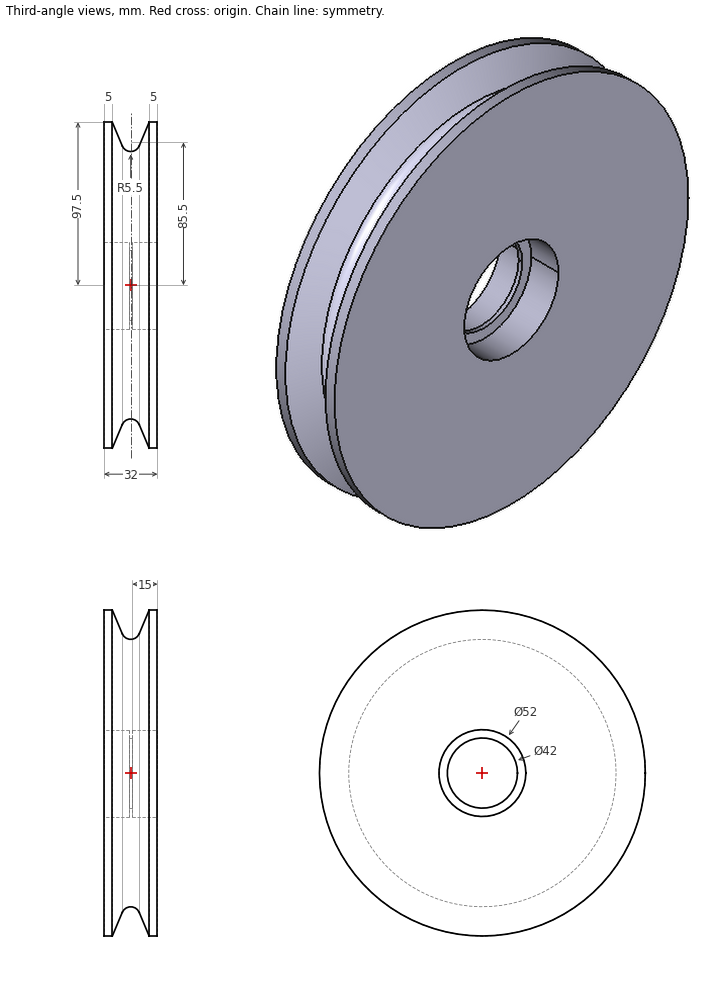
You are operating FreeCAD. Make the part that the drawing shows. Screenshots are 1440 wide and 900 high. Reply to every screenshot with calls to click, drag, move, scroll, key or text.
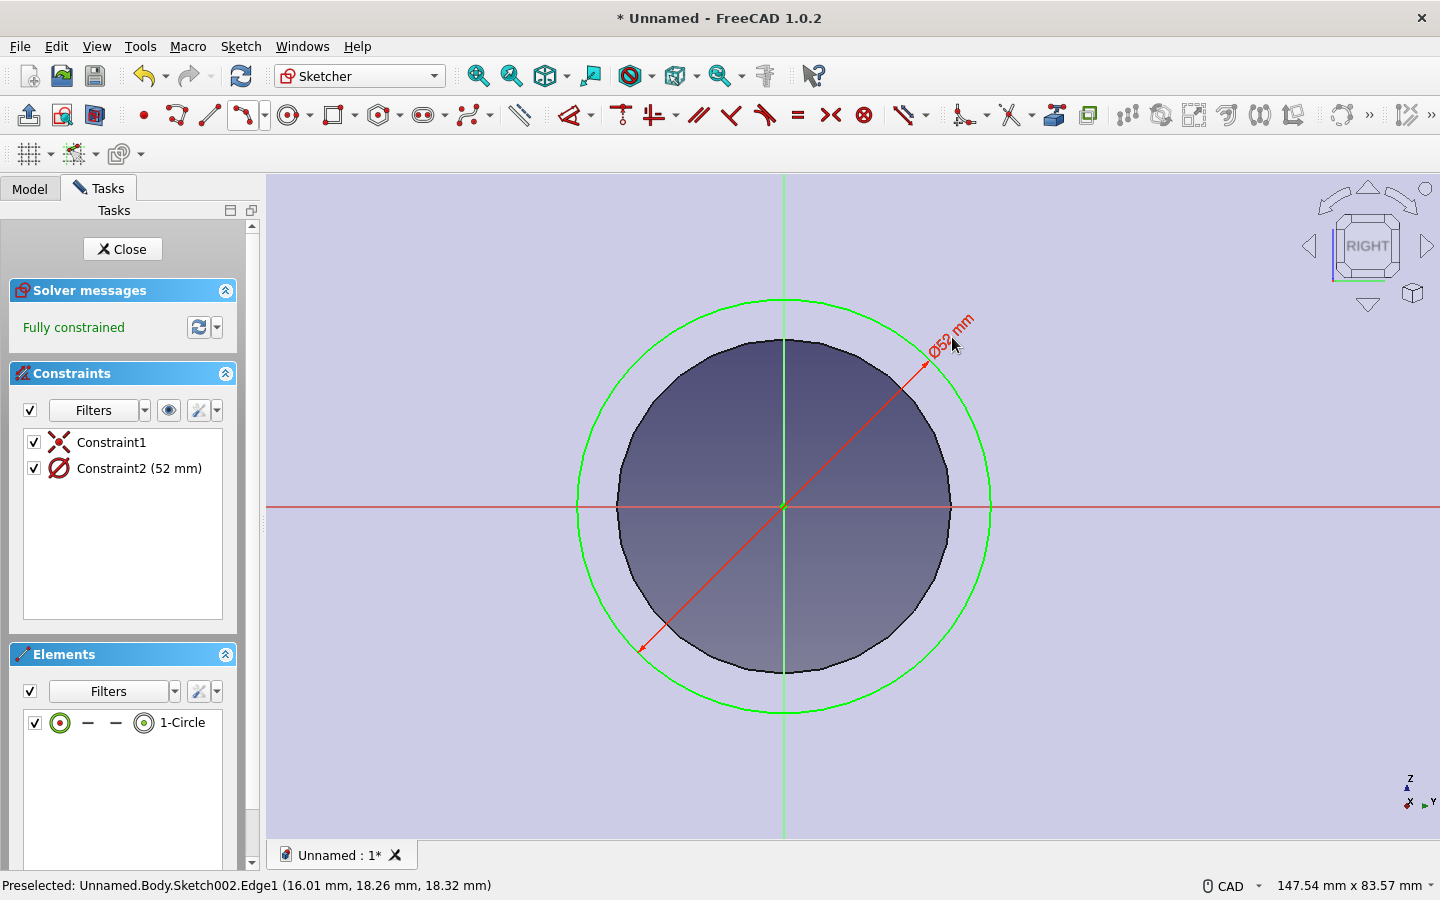
click(123, 249)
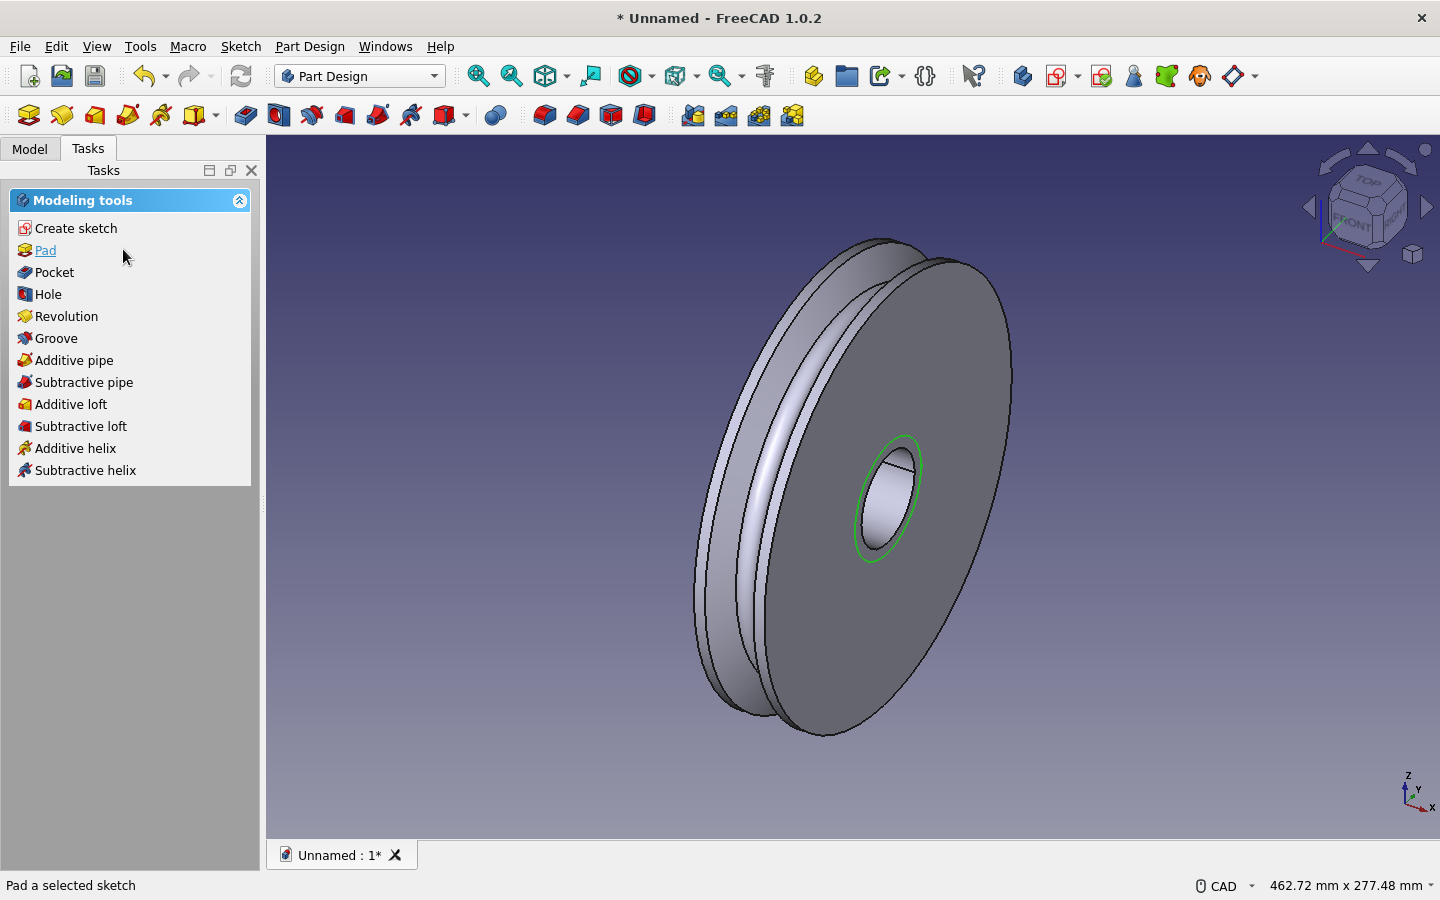
click(246, 116)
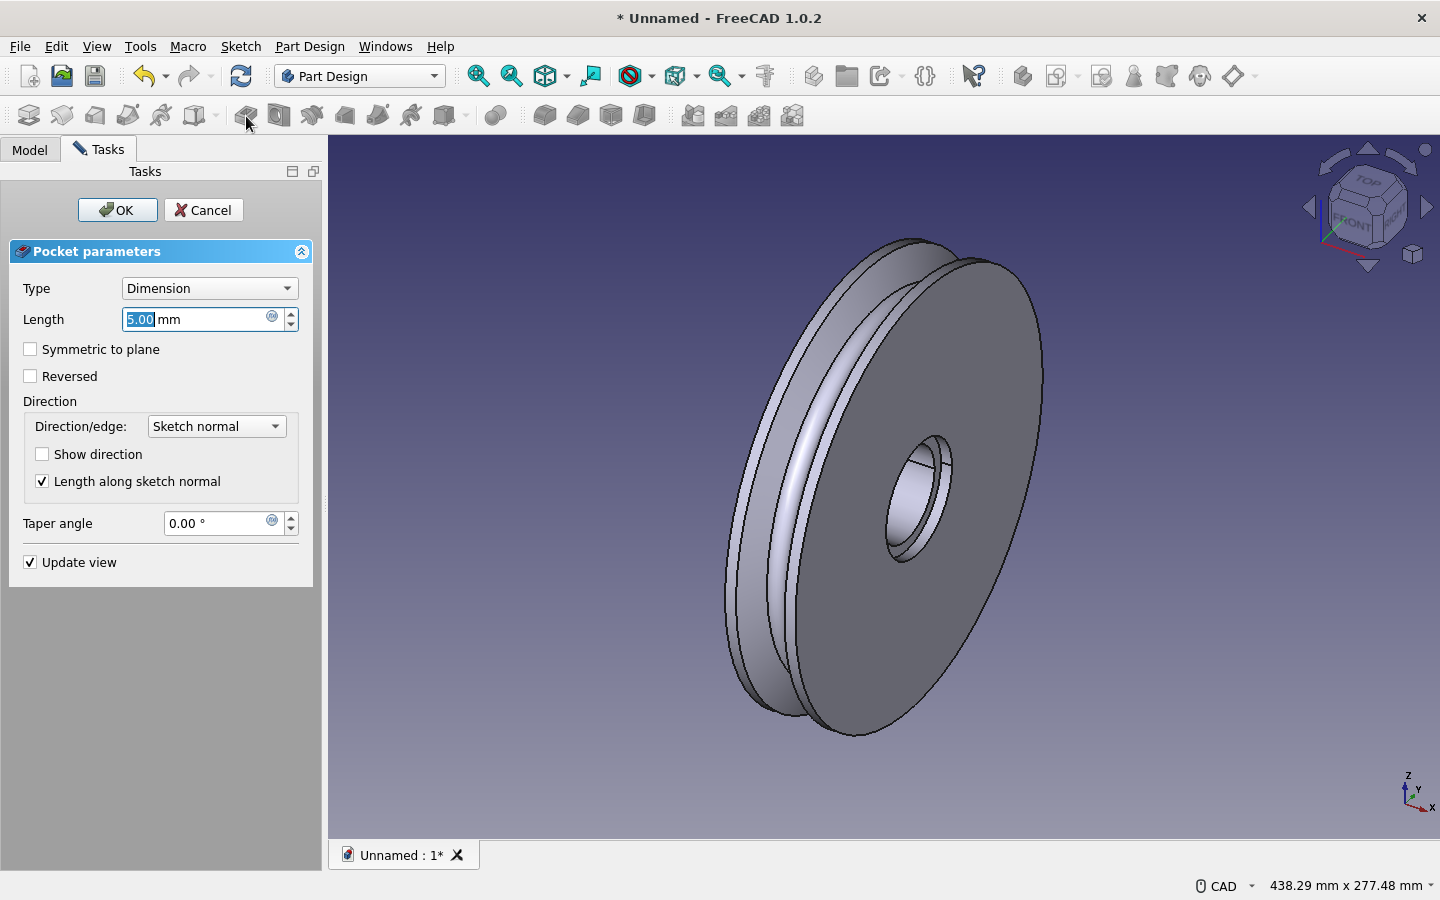
text(15)
key(Tab)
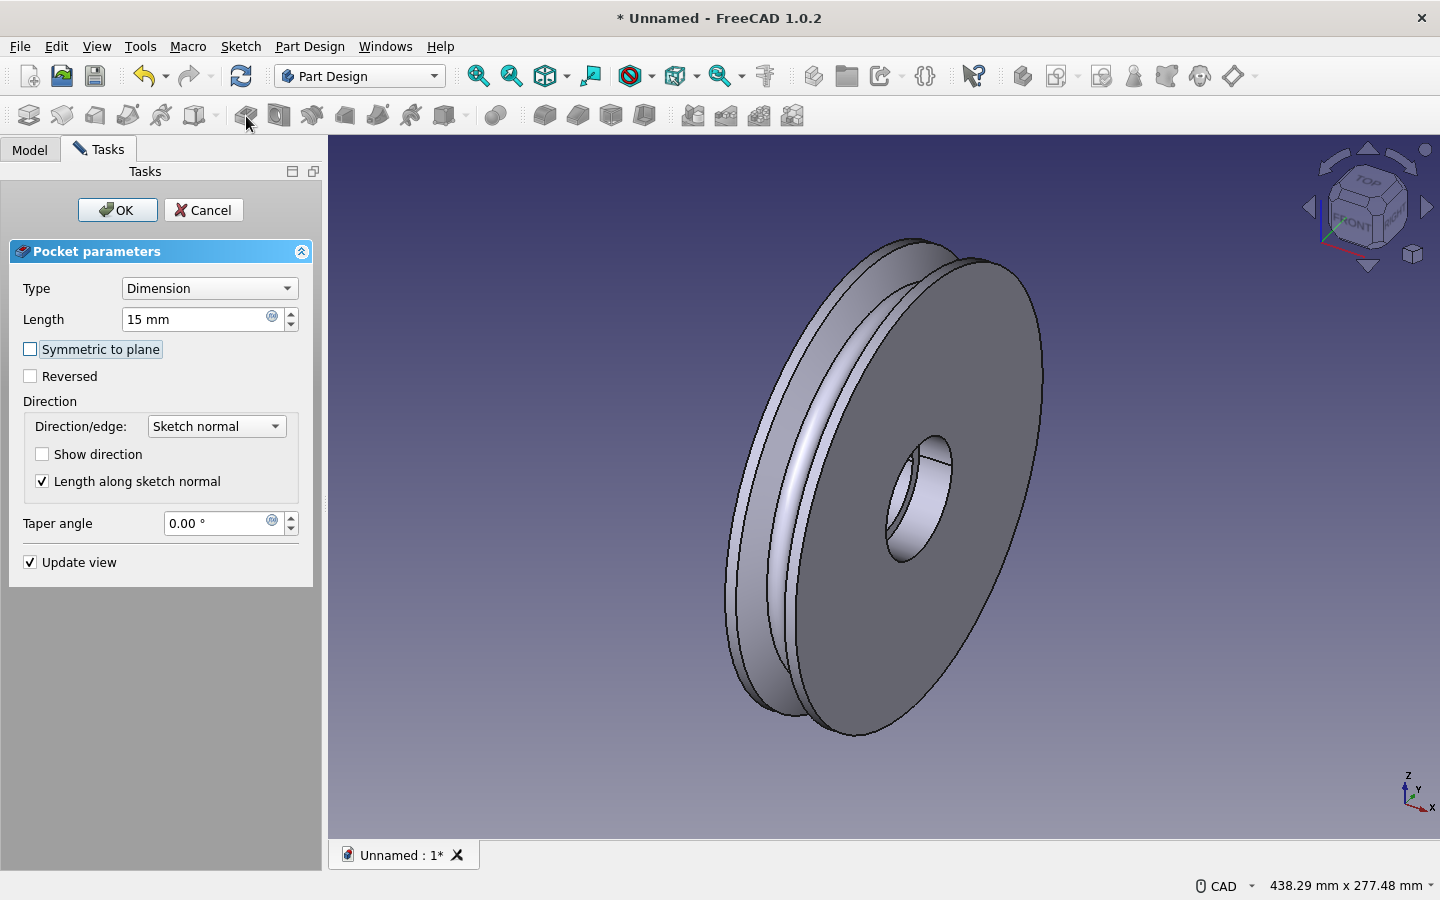
click(118, 210)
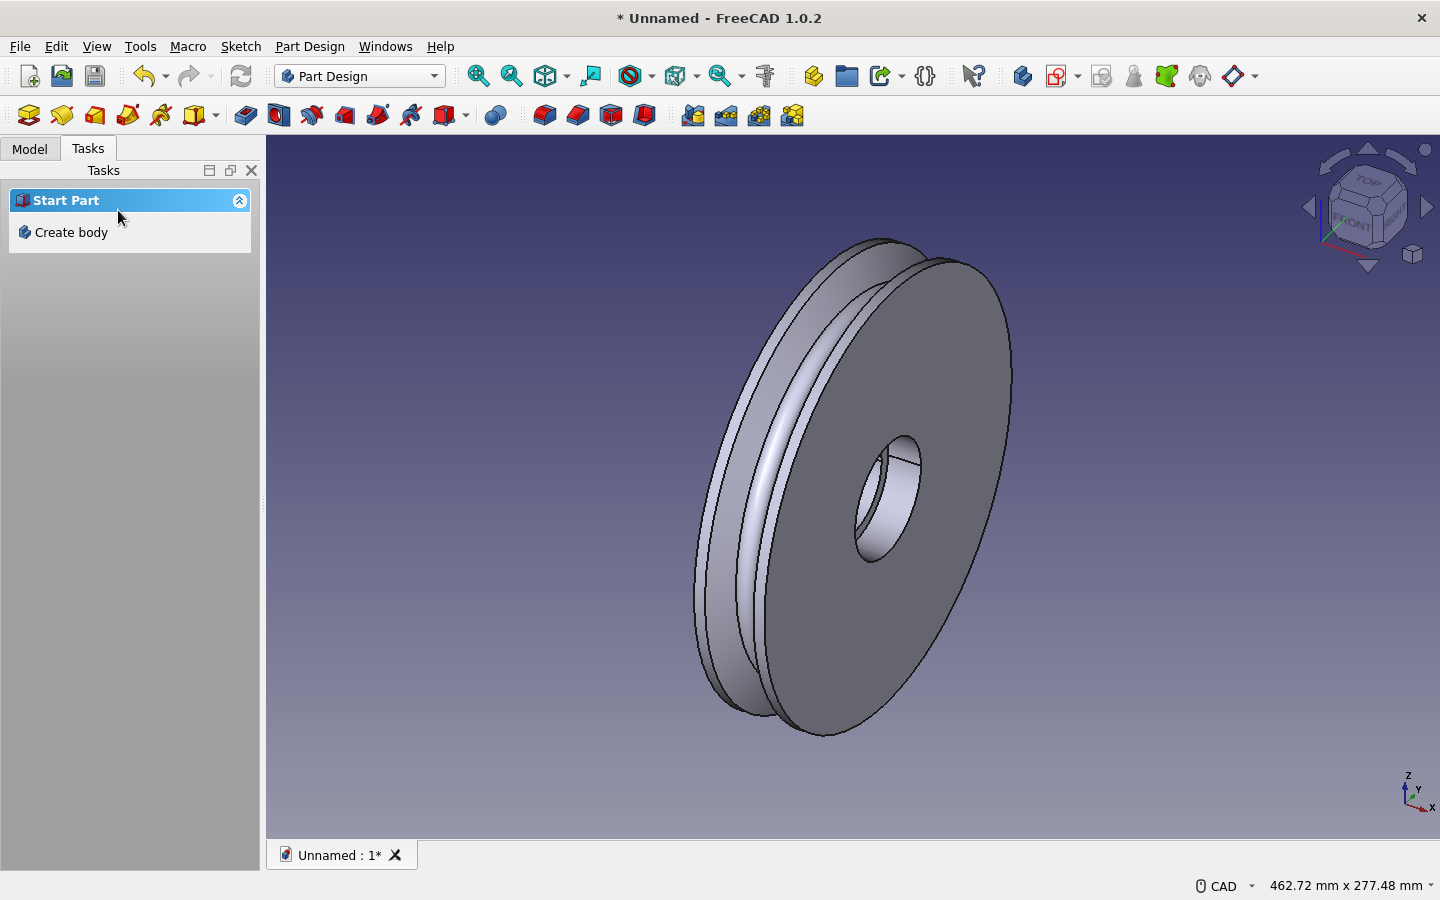
click(30, 148)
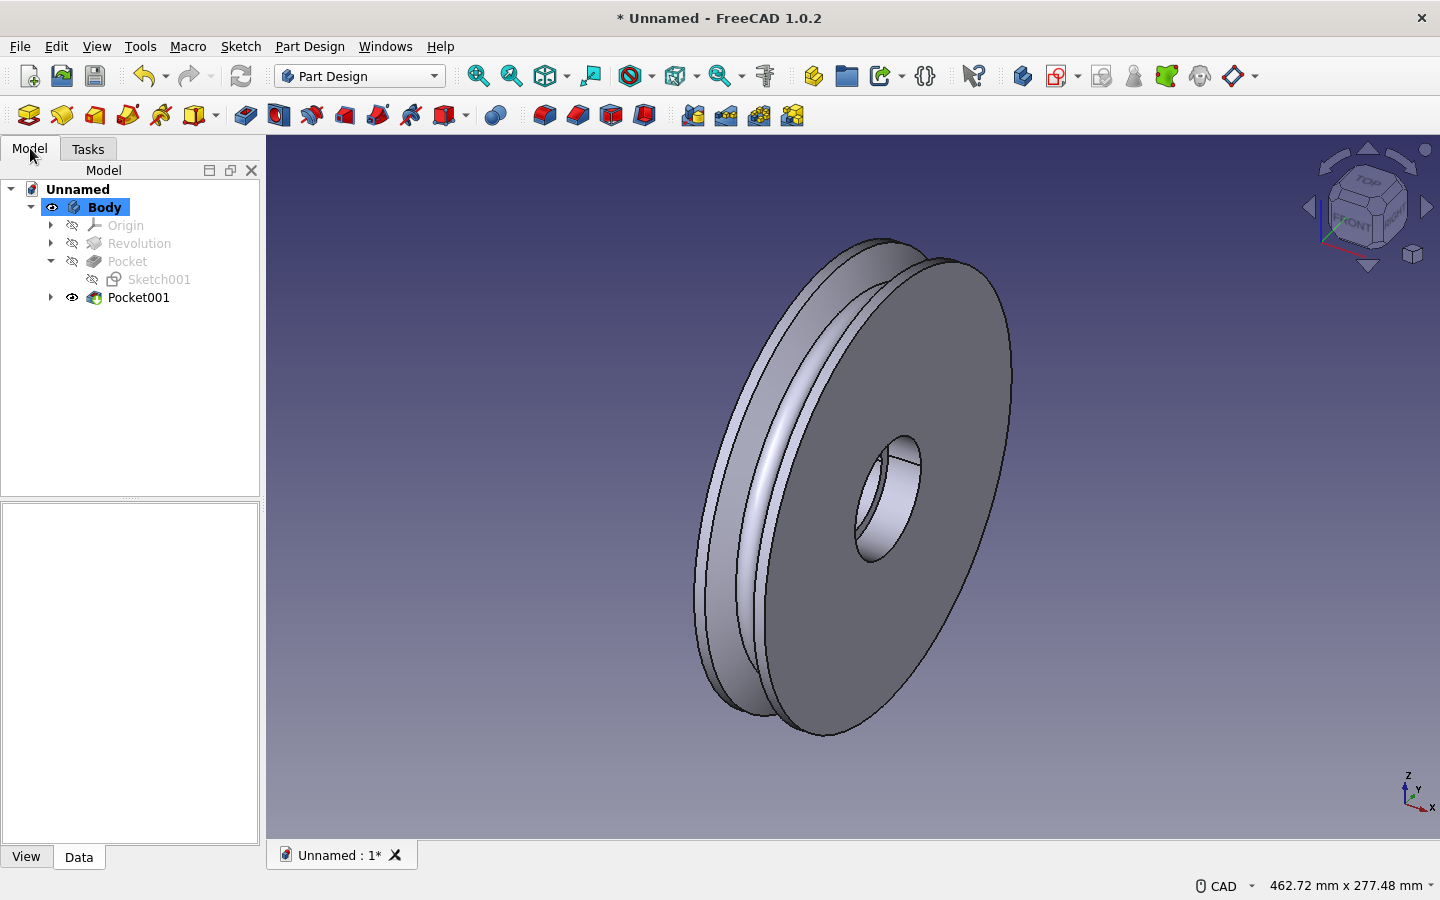
click(117, 297)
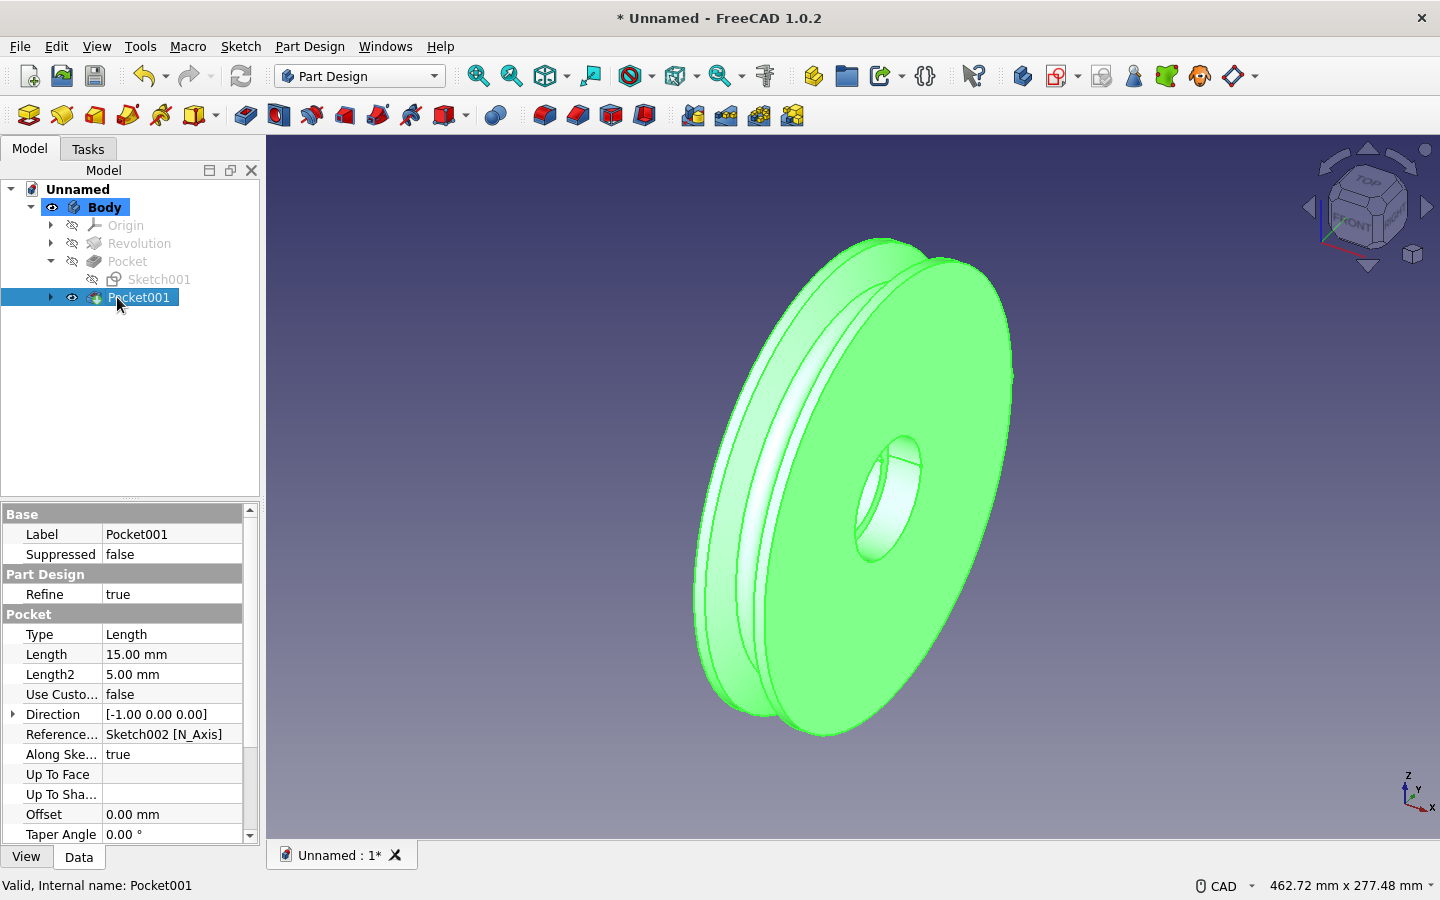
click(693, 116)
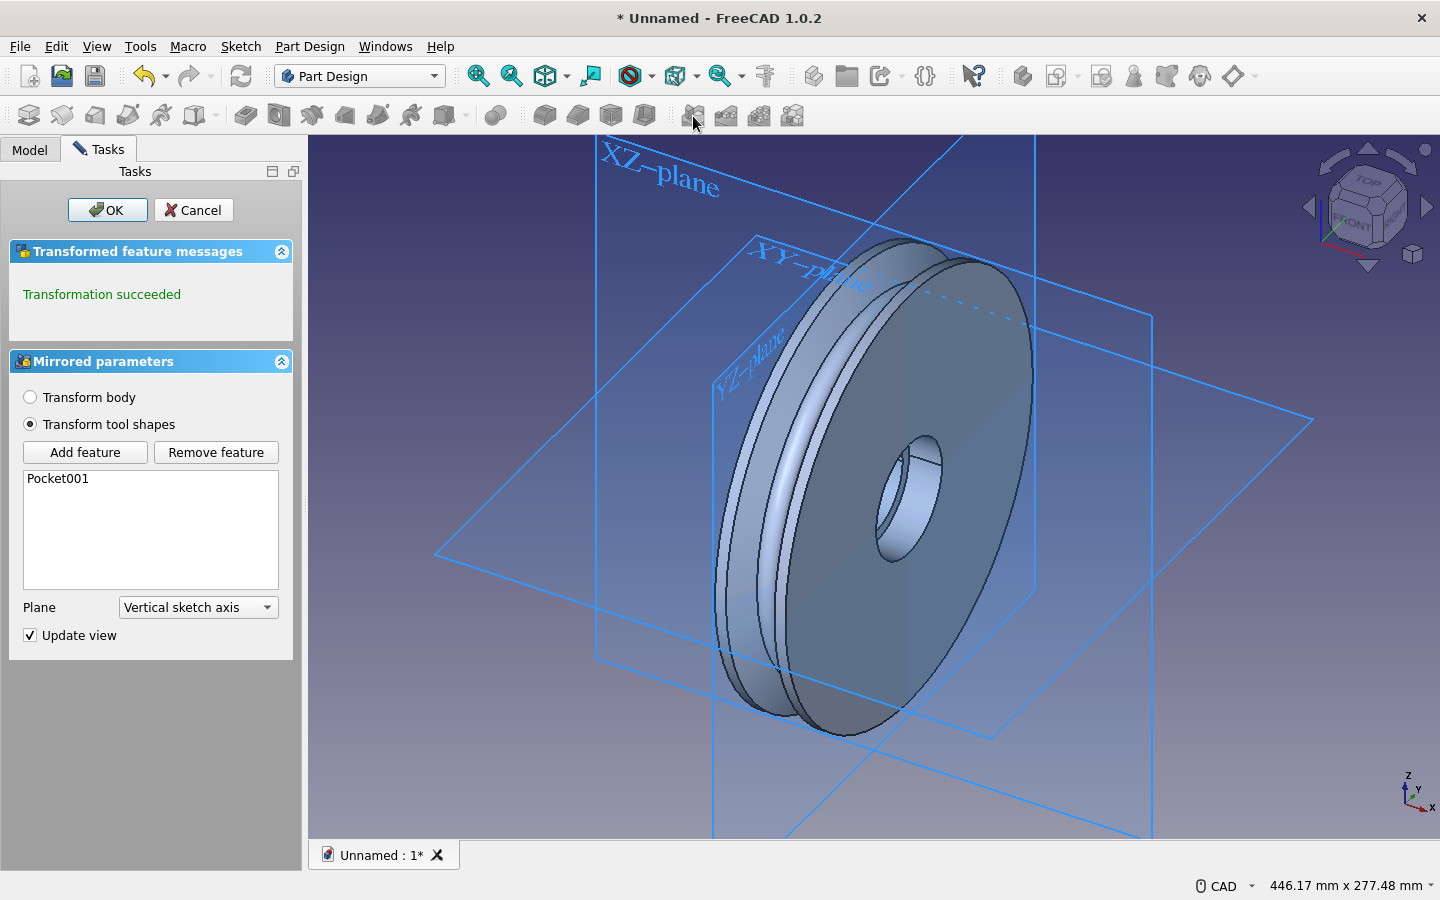
click(199, 608)